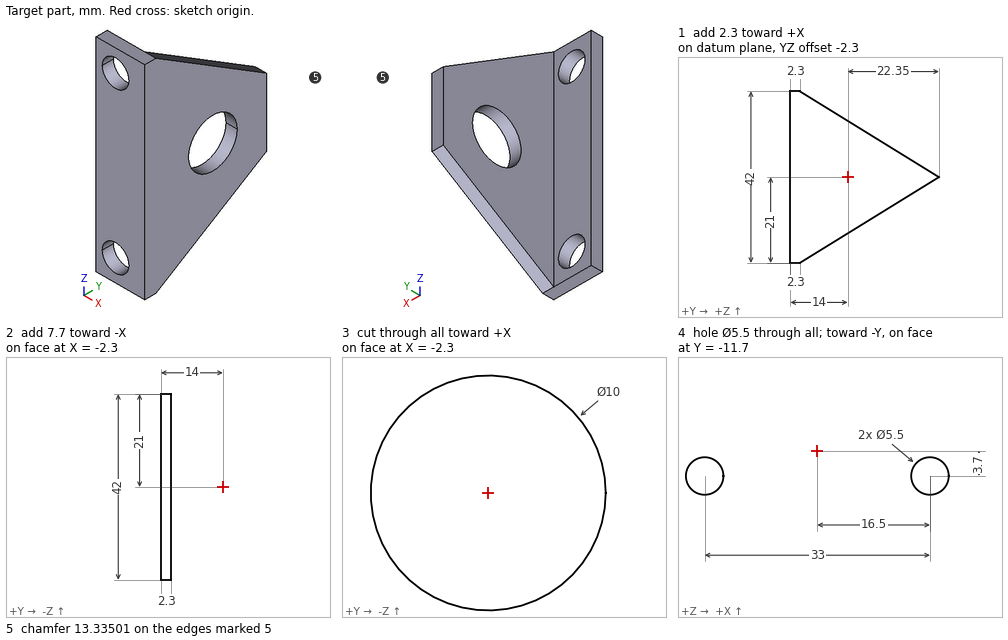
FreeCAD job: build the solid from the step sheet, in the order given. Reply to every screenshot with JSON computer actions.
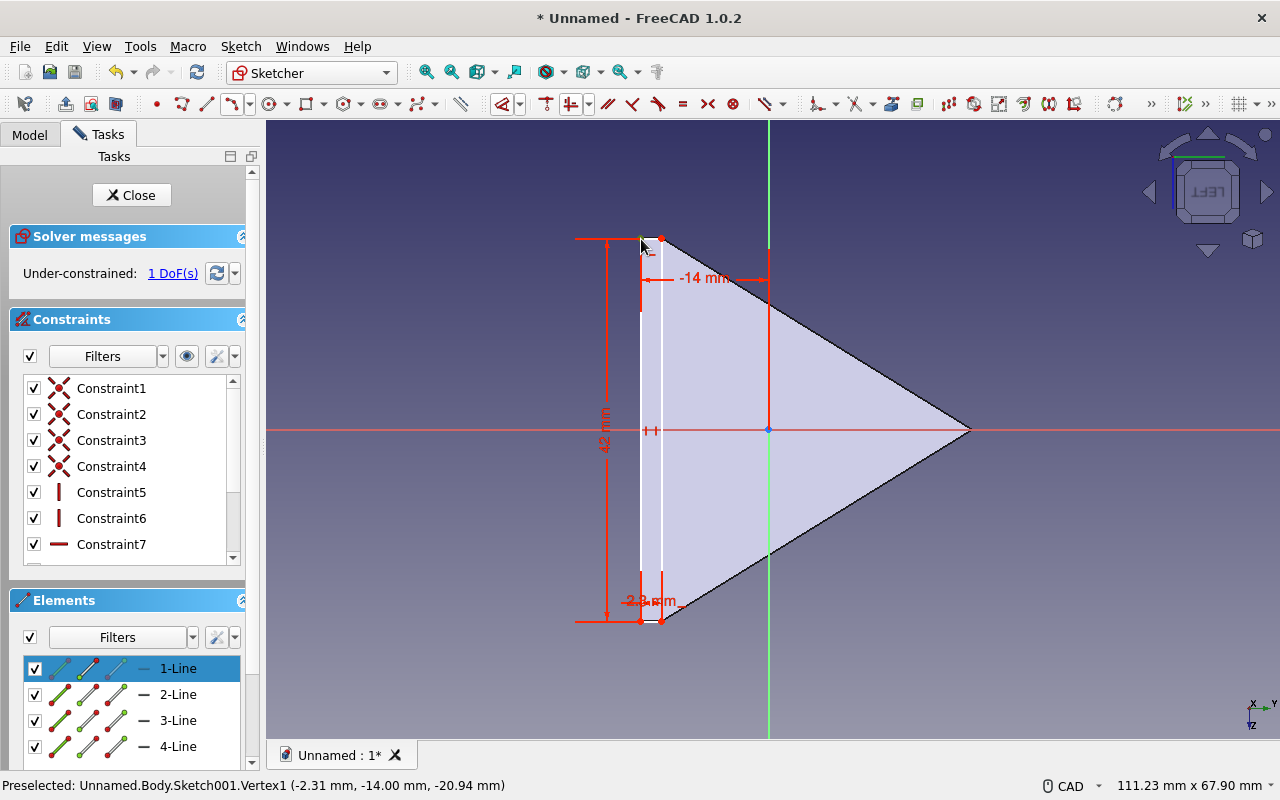
{"action": "key", "text": "i"}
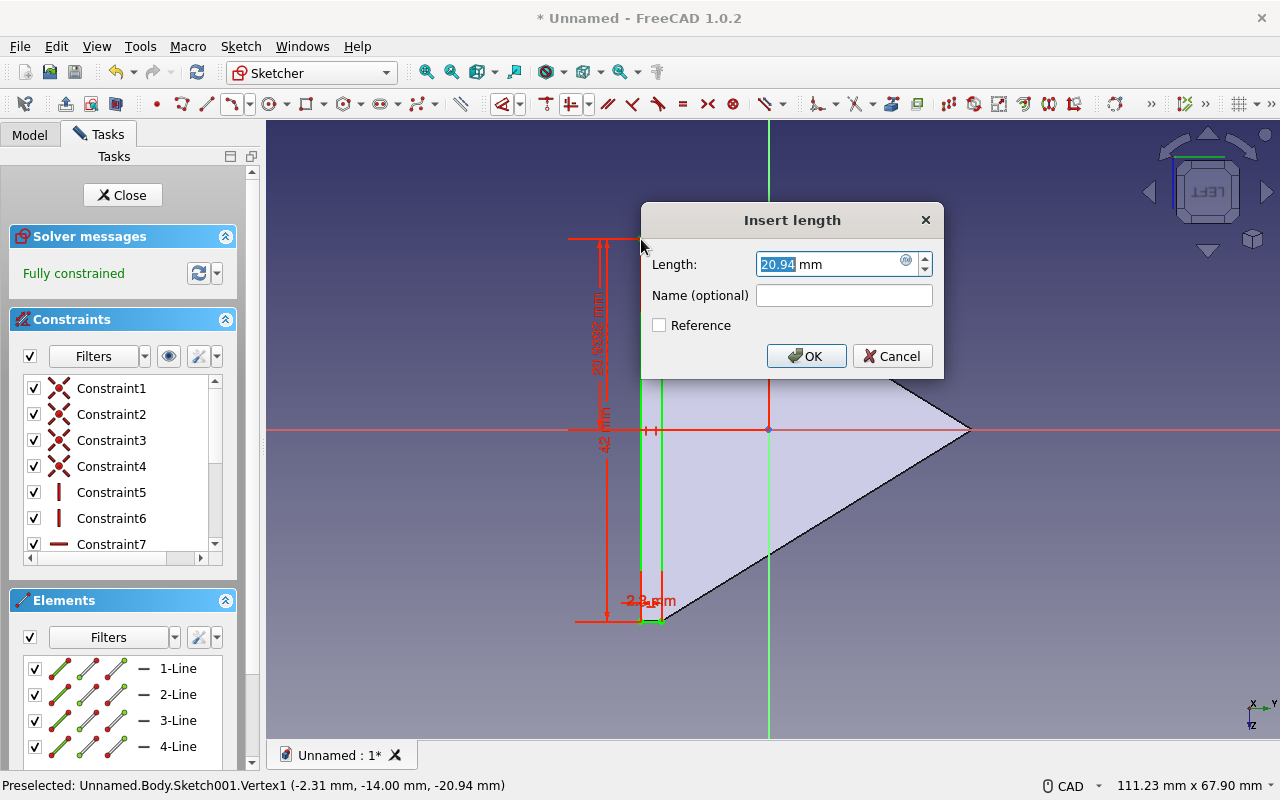
{"action": "type", "text": "21"}
{"action": "key", "text": "Return"}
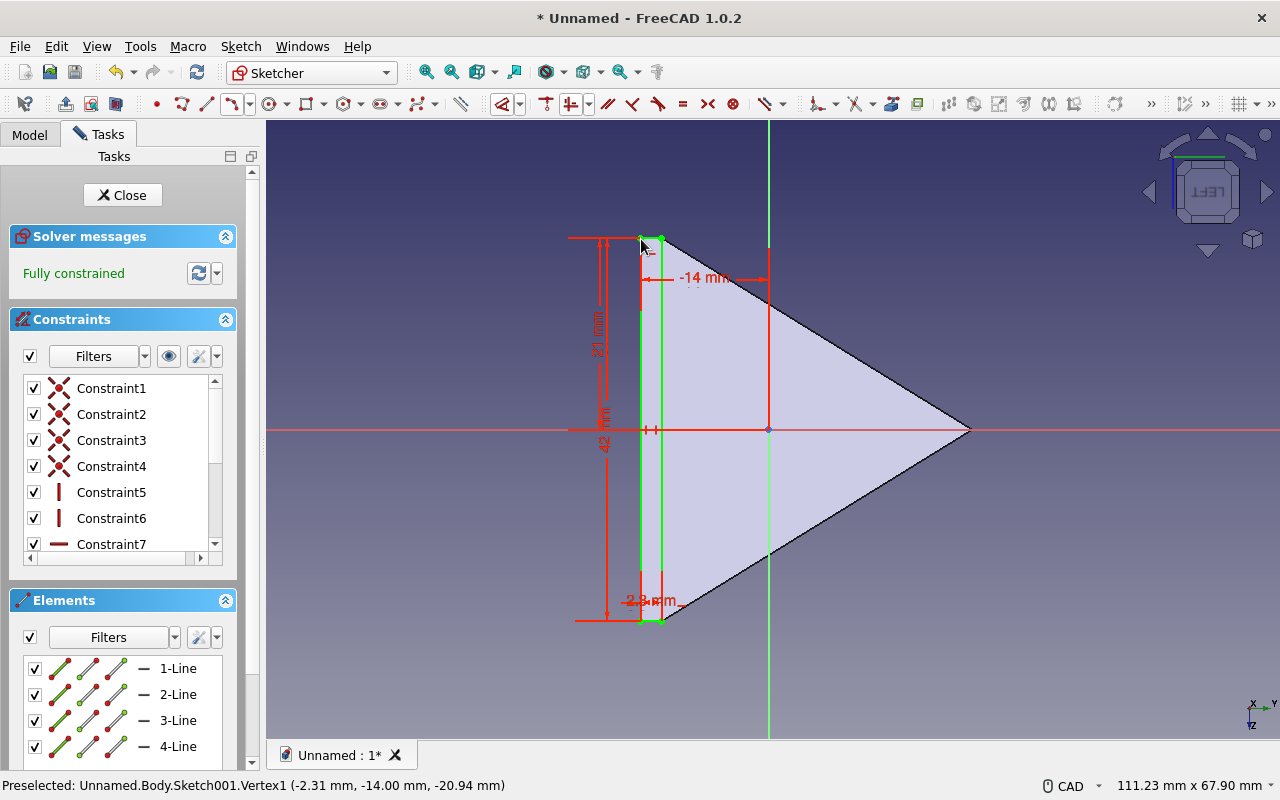
{"action": "left_click", "coordinate": [123, 195]}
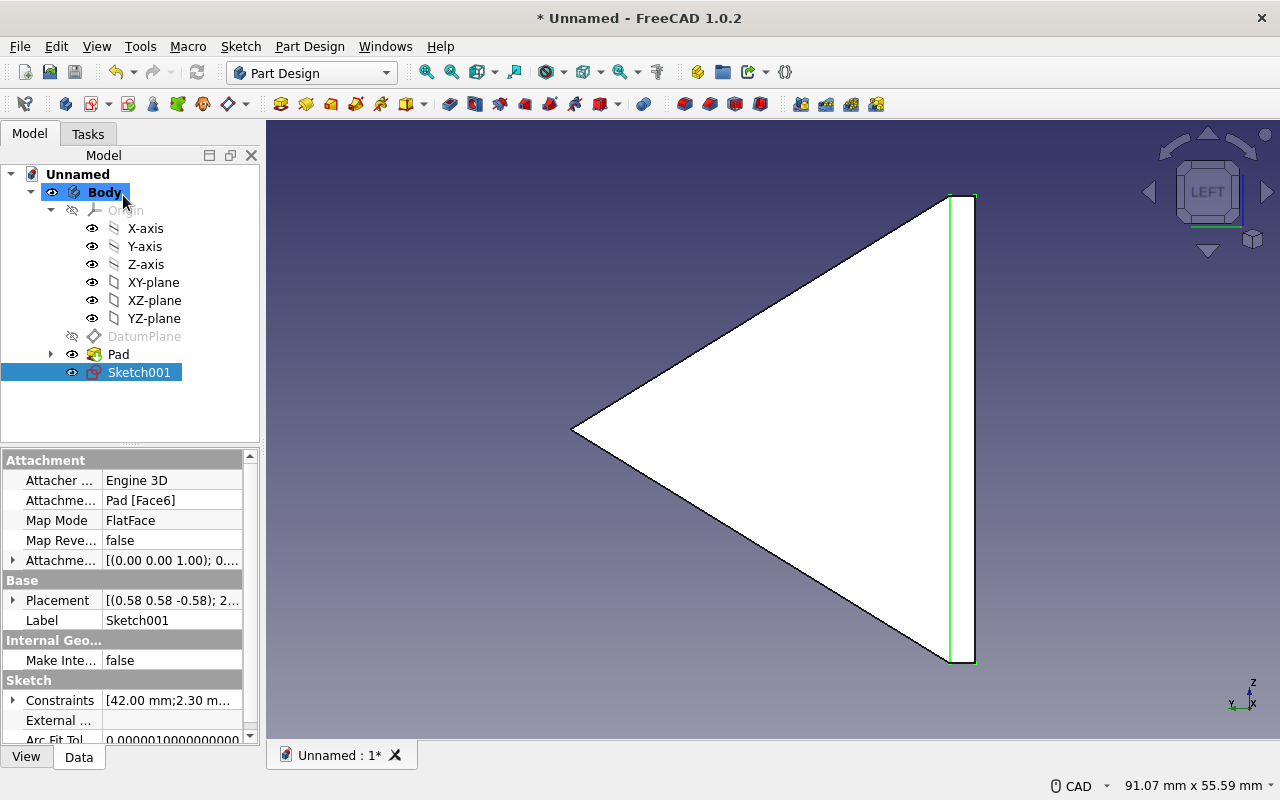
{"action": "left_click", "coordinate": [281, 104]}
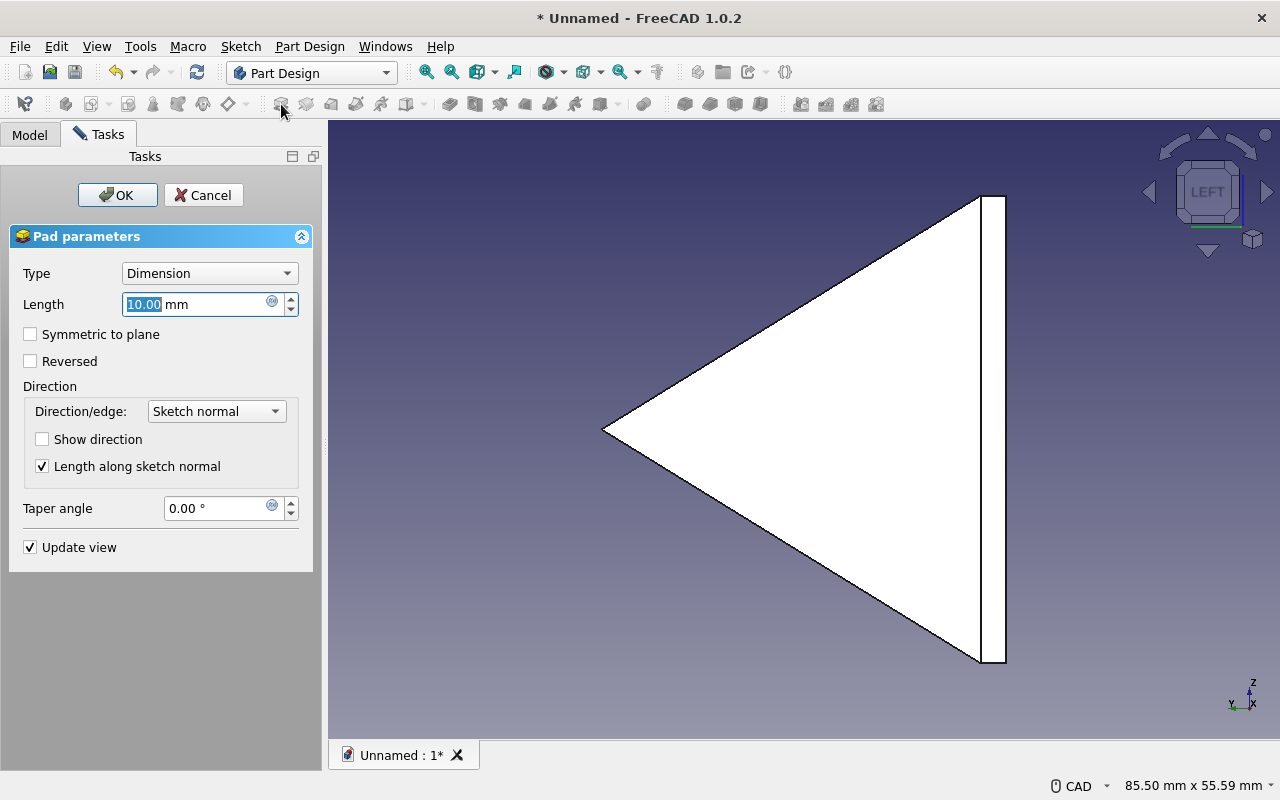
{"action": "type", "text": "7.7"}
{"action": "key", "text": "Tab"}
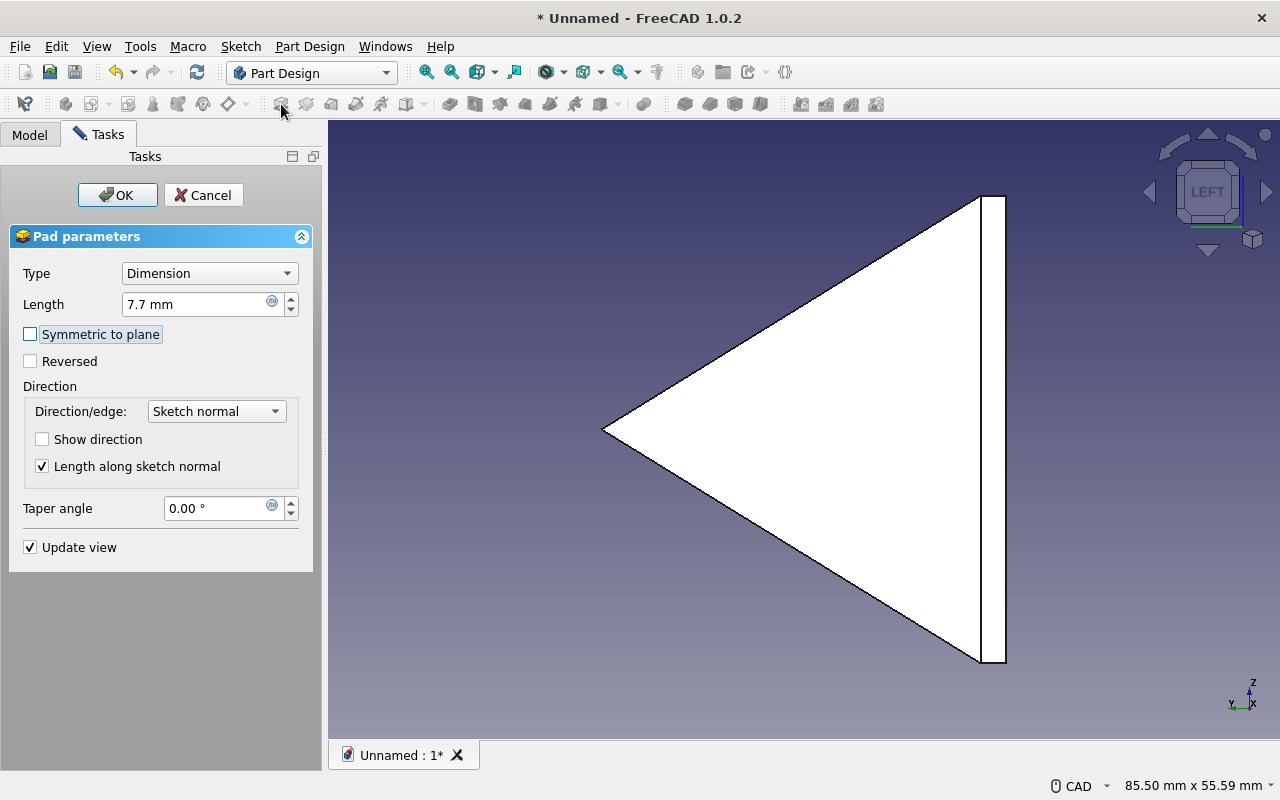
{"action": "left_click", "coordinate": [118, 195]}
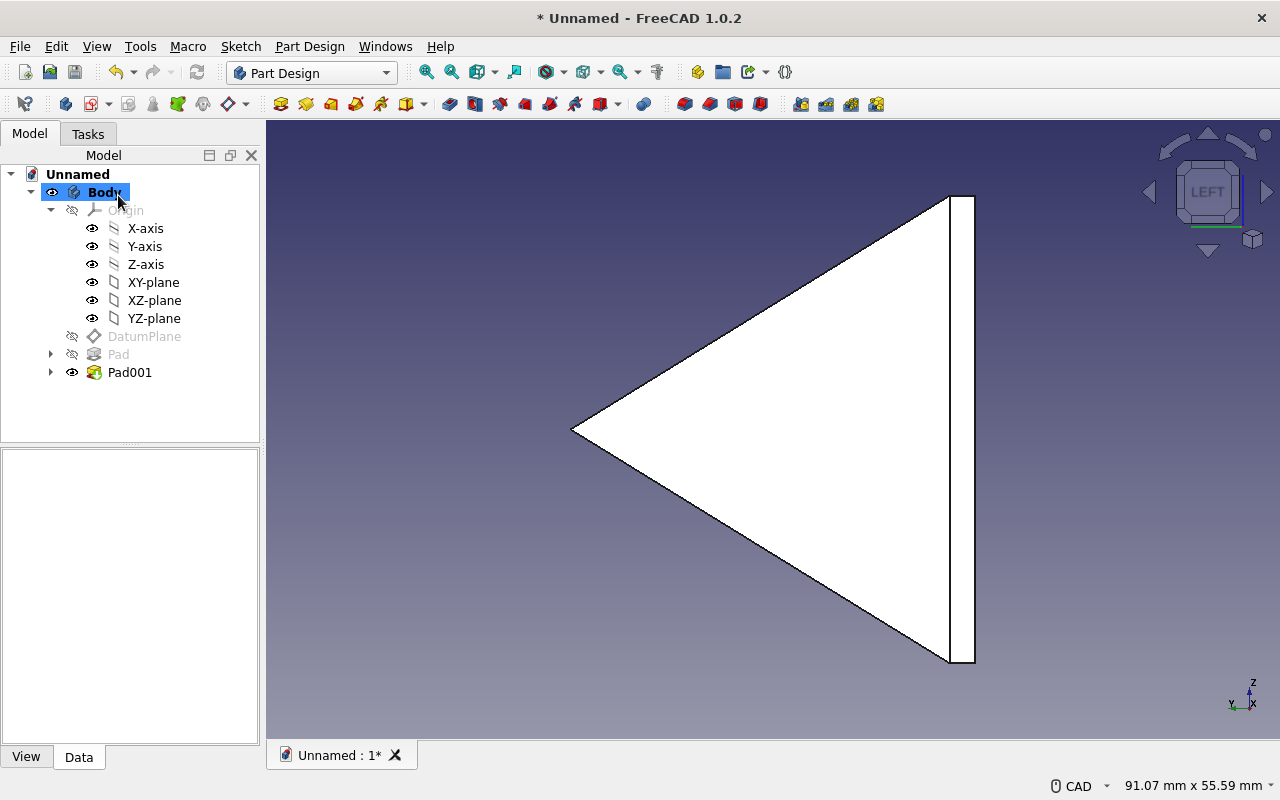
{"action": "left_click", "coordinate": [814, 428]}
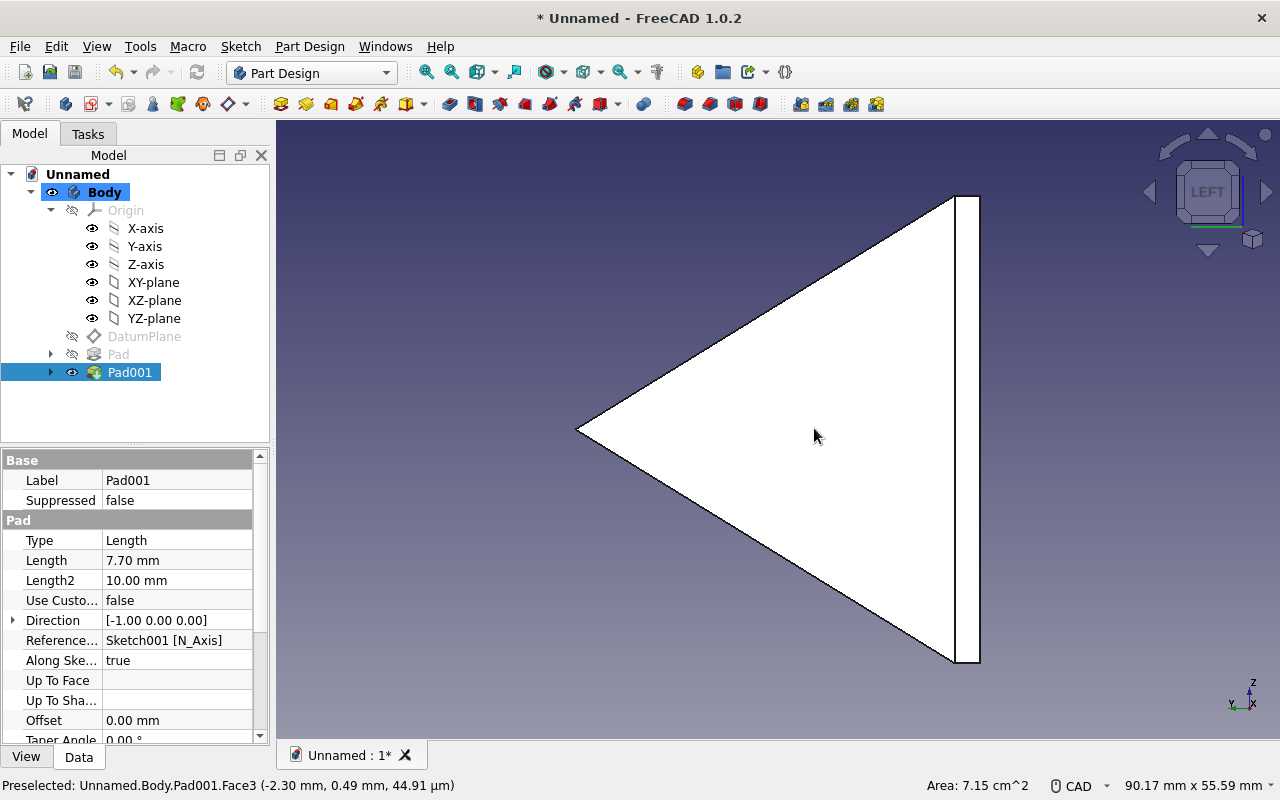
{"action": "left_click", "coordinate": [90, 104]}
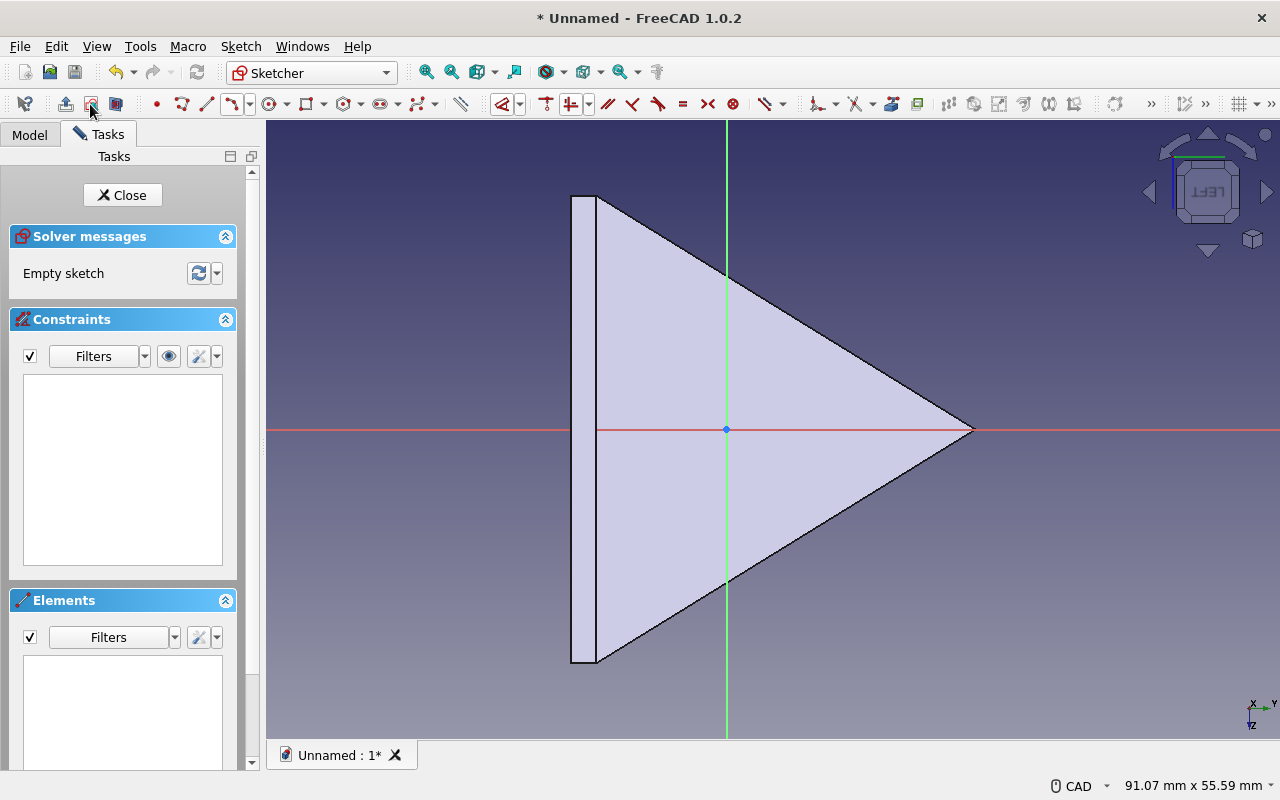
{"action": "scroll", "coordinate": [736, 429], "scroll_direction": "up", "scroll_amount": 6}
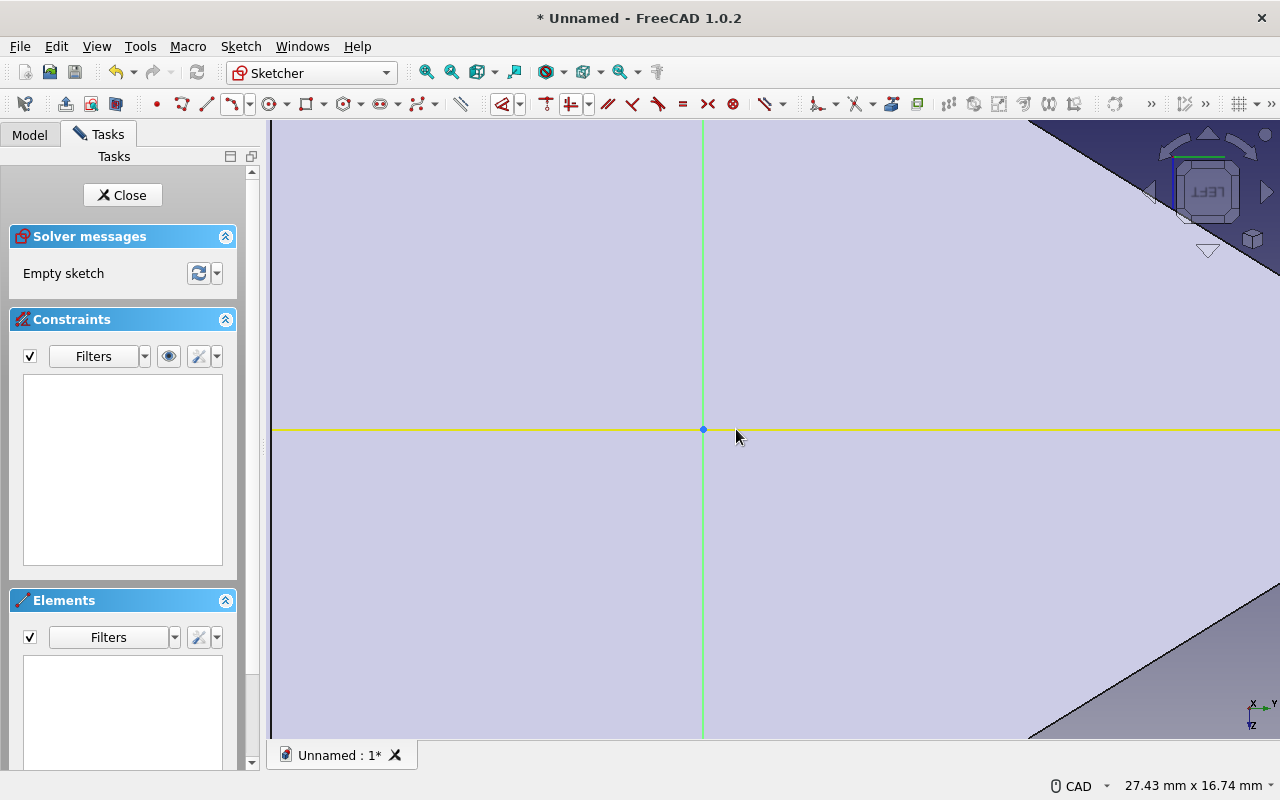
{"action": "key", "text": "g c"}